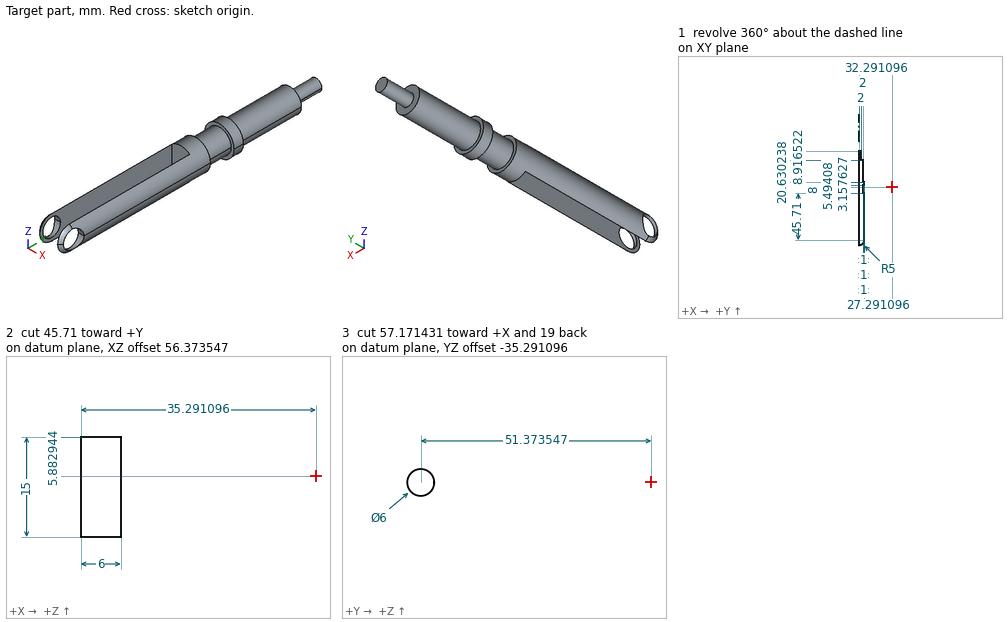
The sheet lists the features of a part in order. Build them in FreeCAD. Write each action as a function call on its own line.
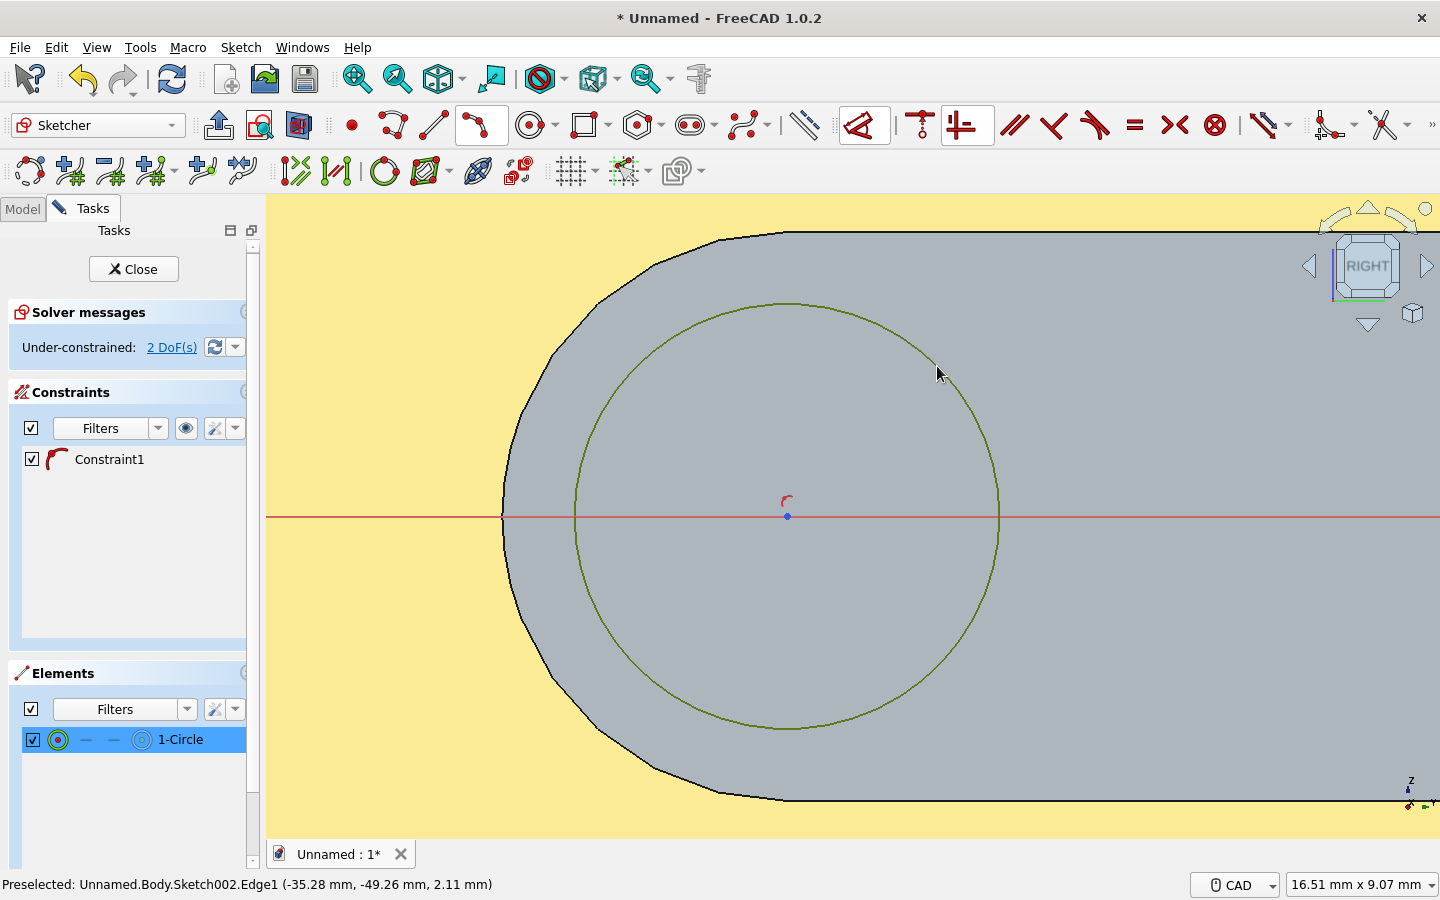
key(k)
key(o)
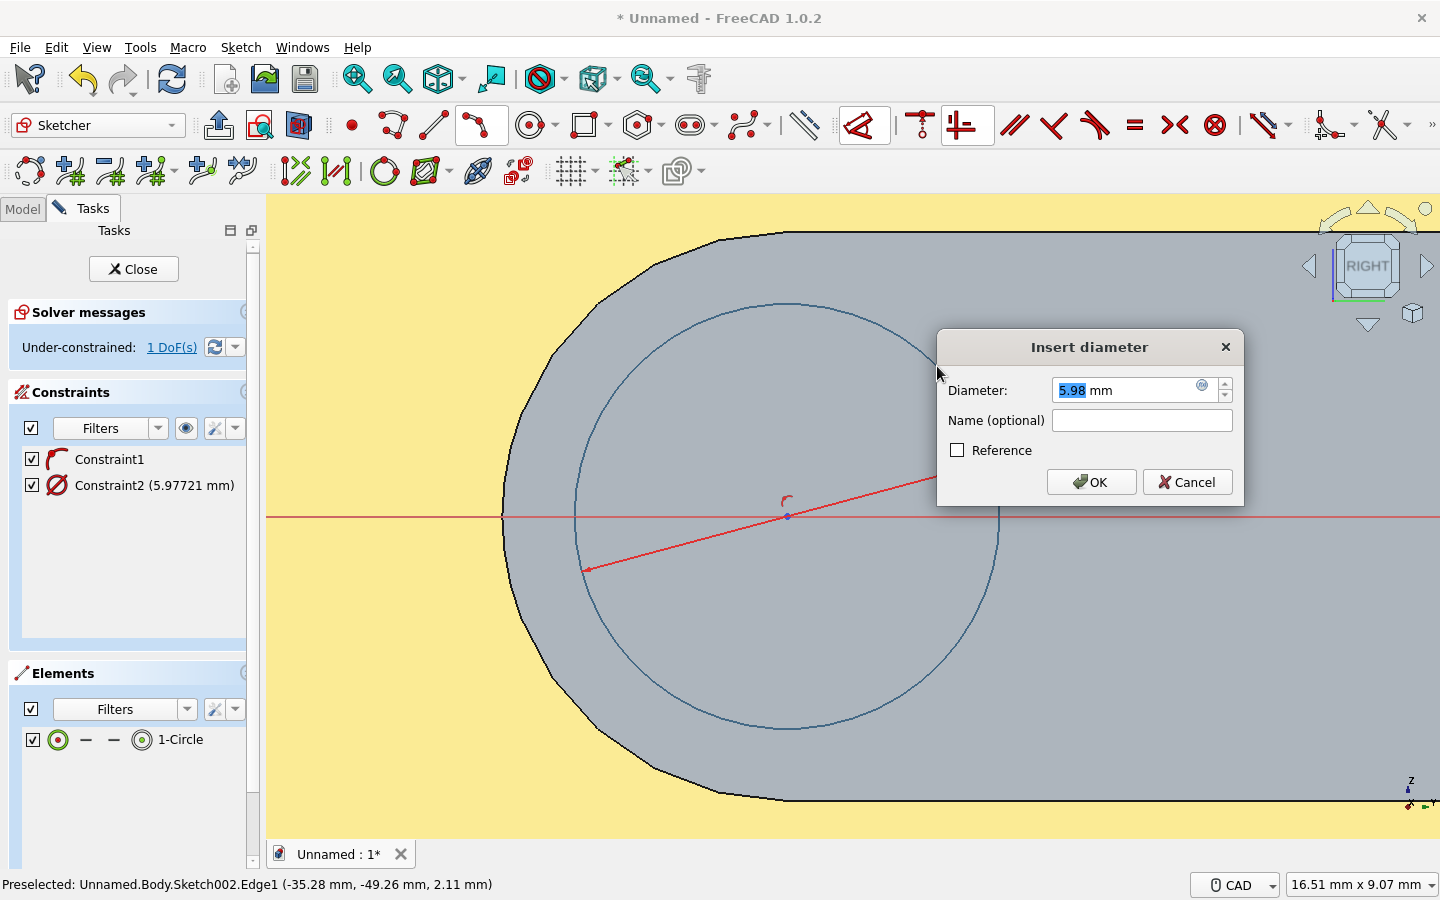
text(6)
key(Return)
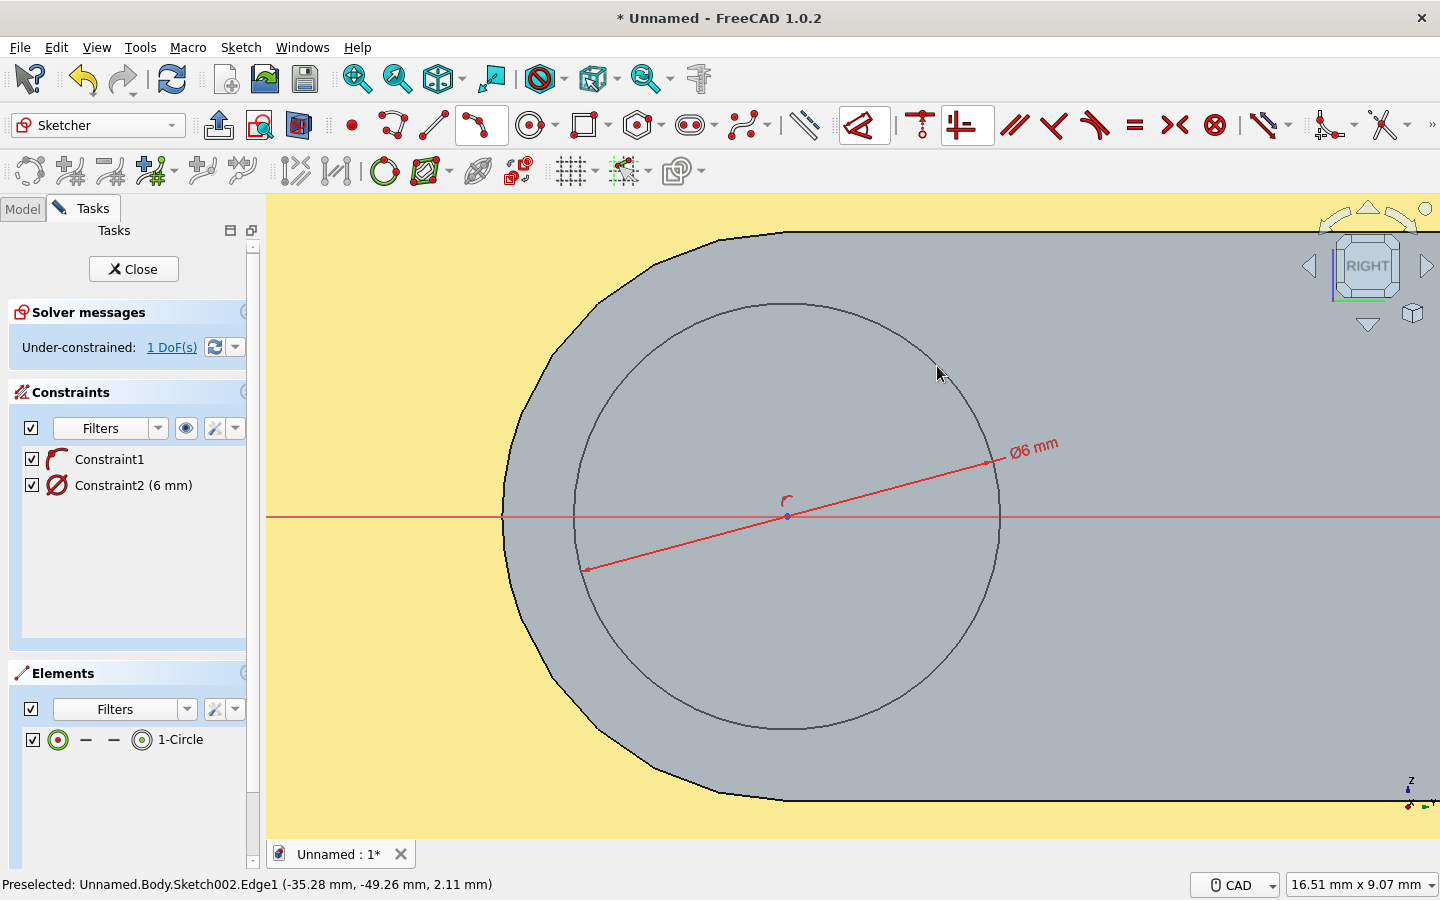
click(787, 516)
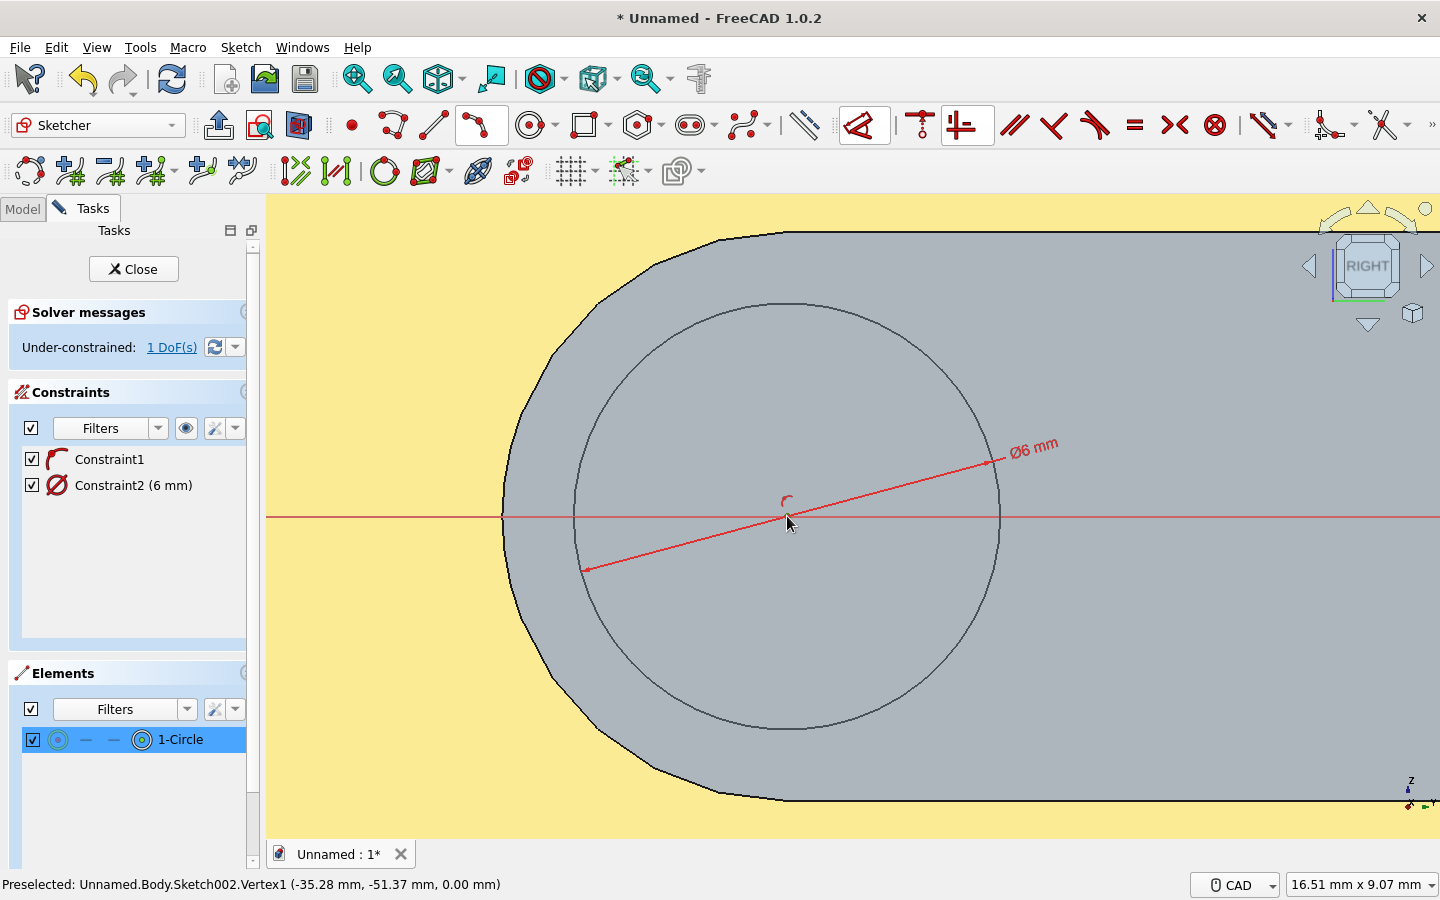
click(884, 126)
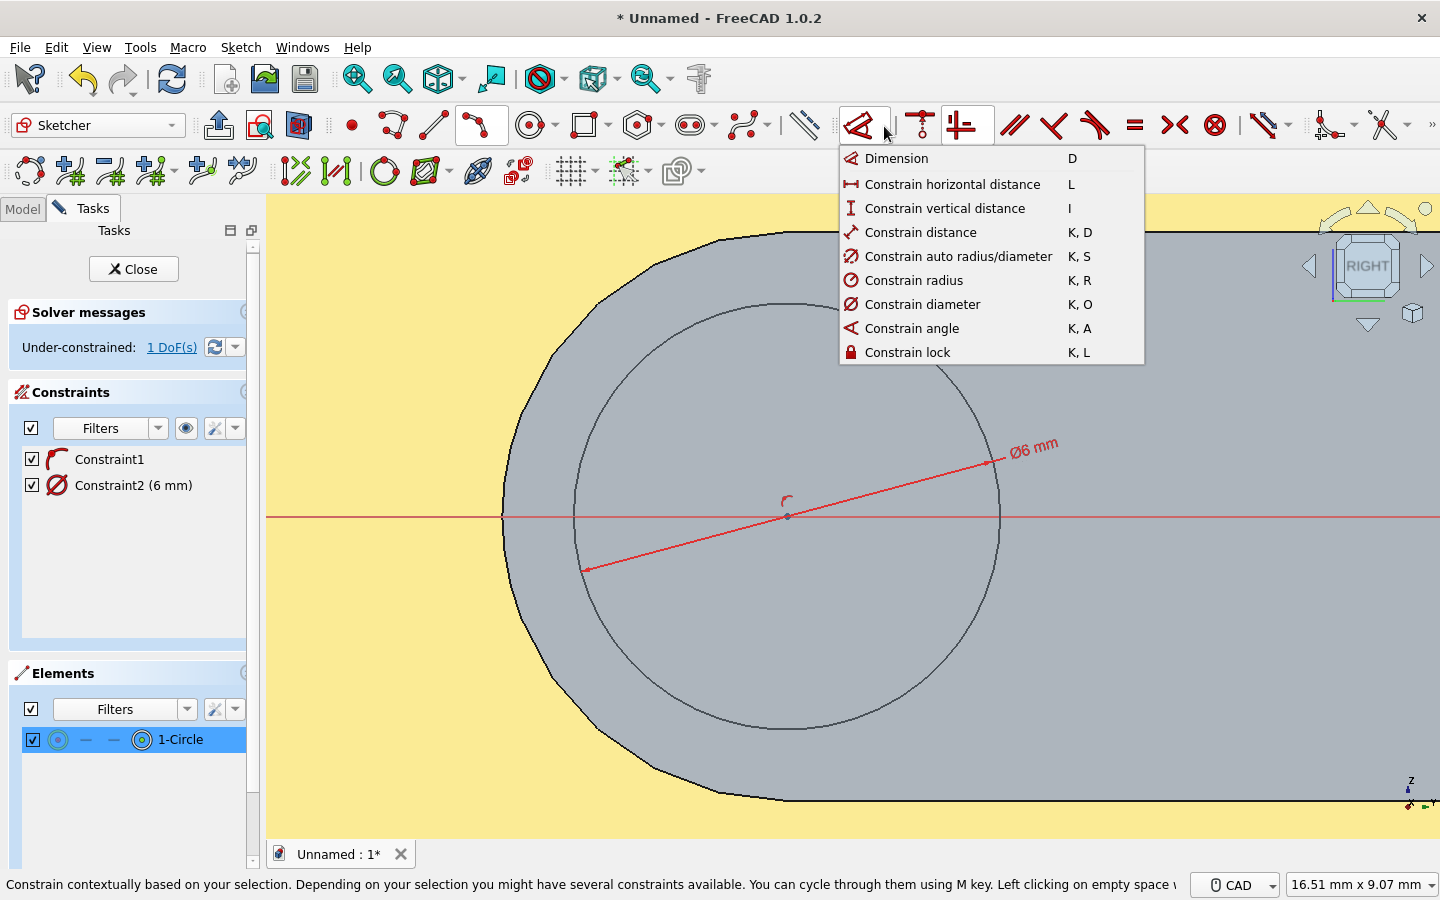
click(992, 184)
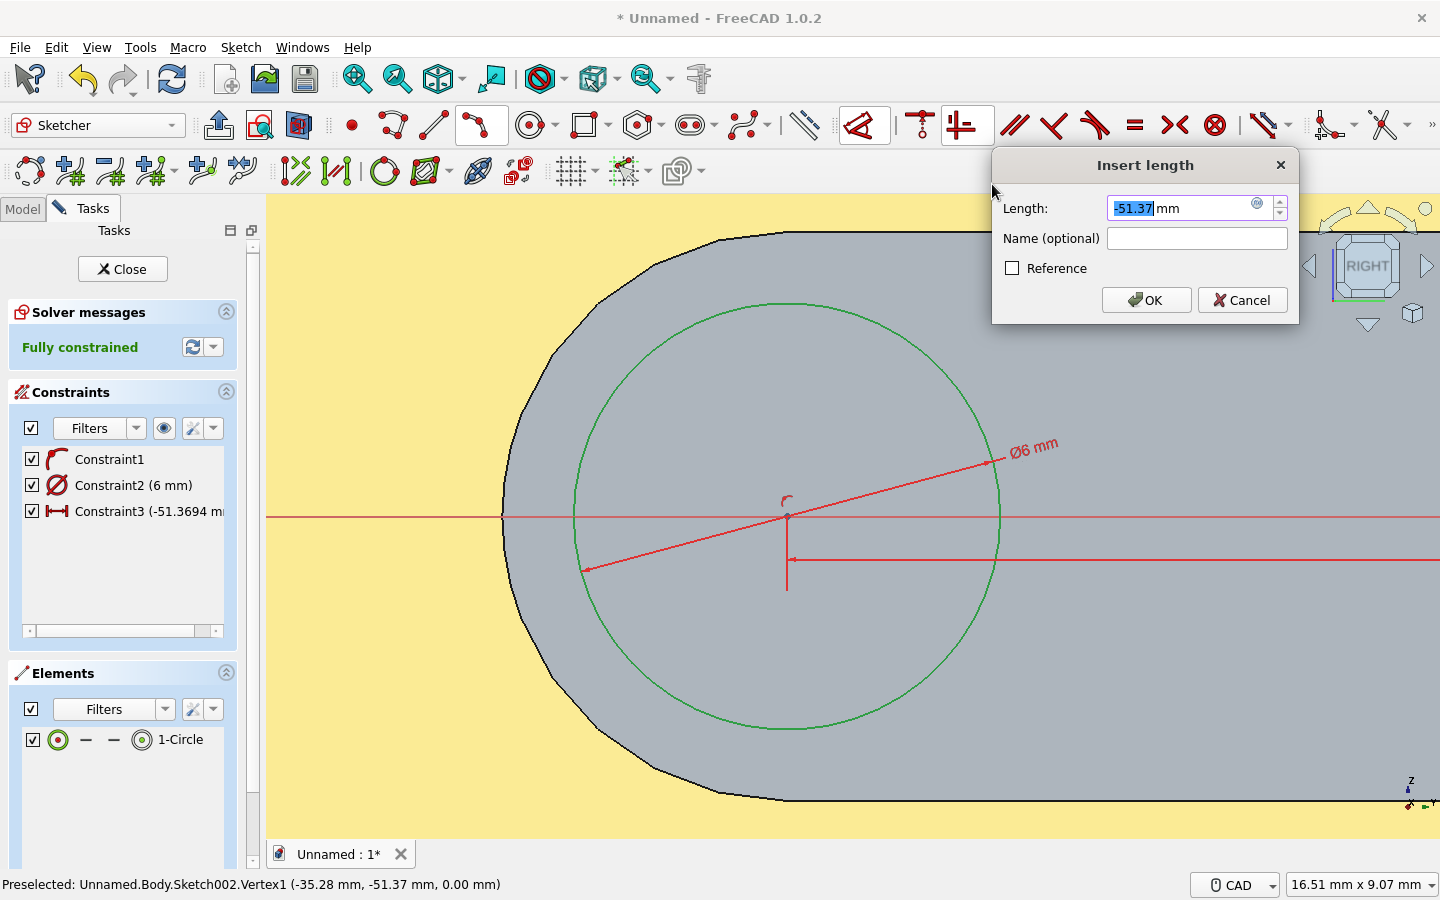
text(-51.373547)
key(Return)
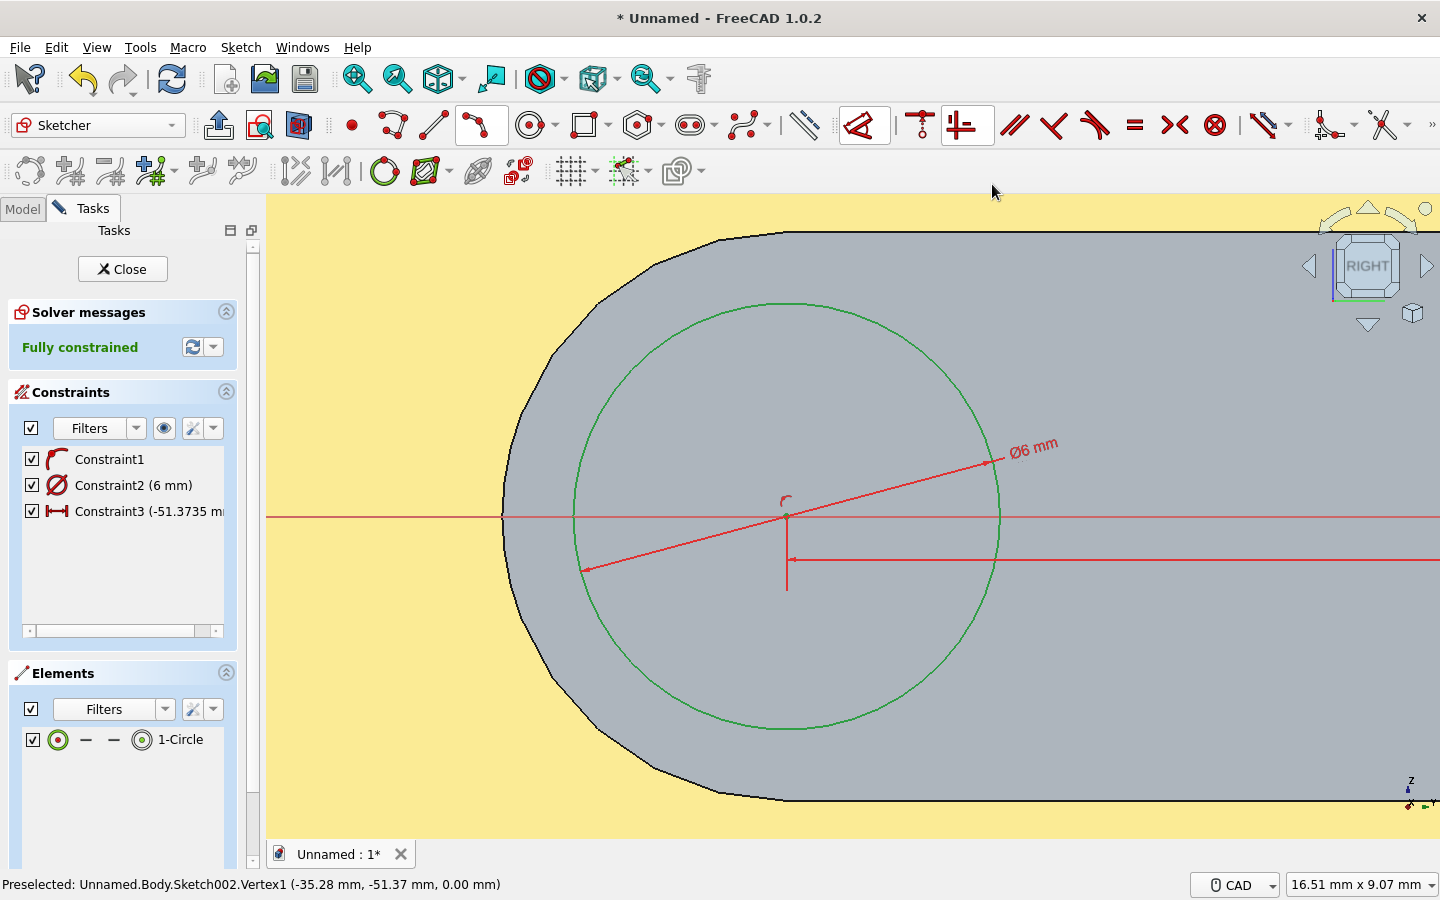
click(123, 269)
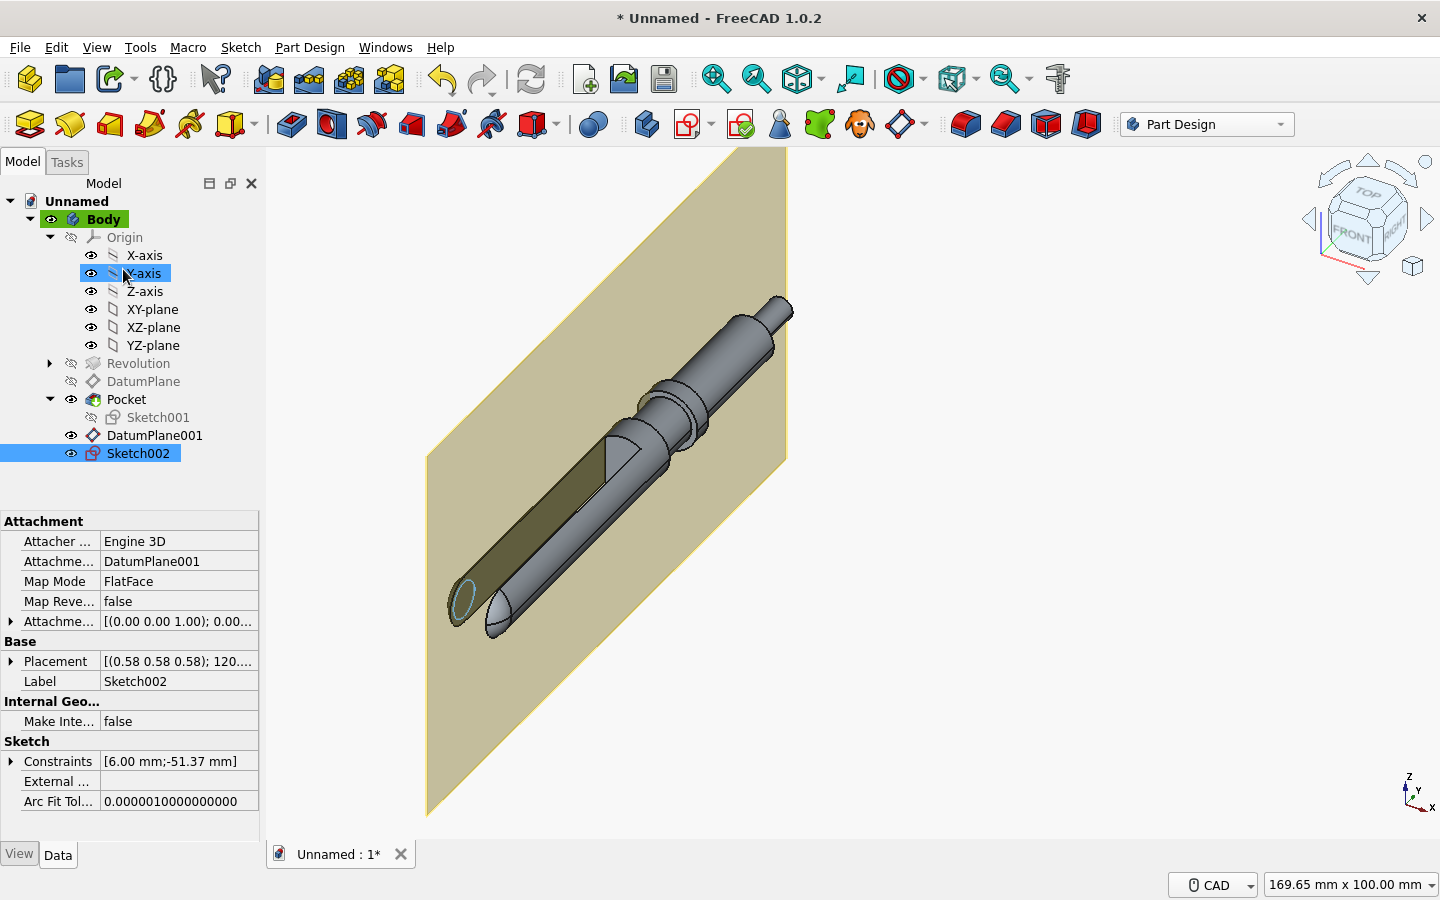
click(292, 124)